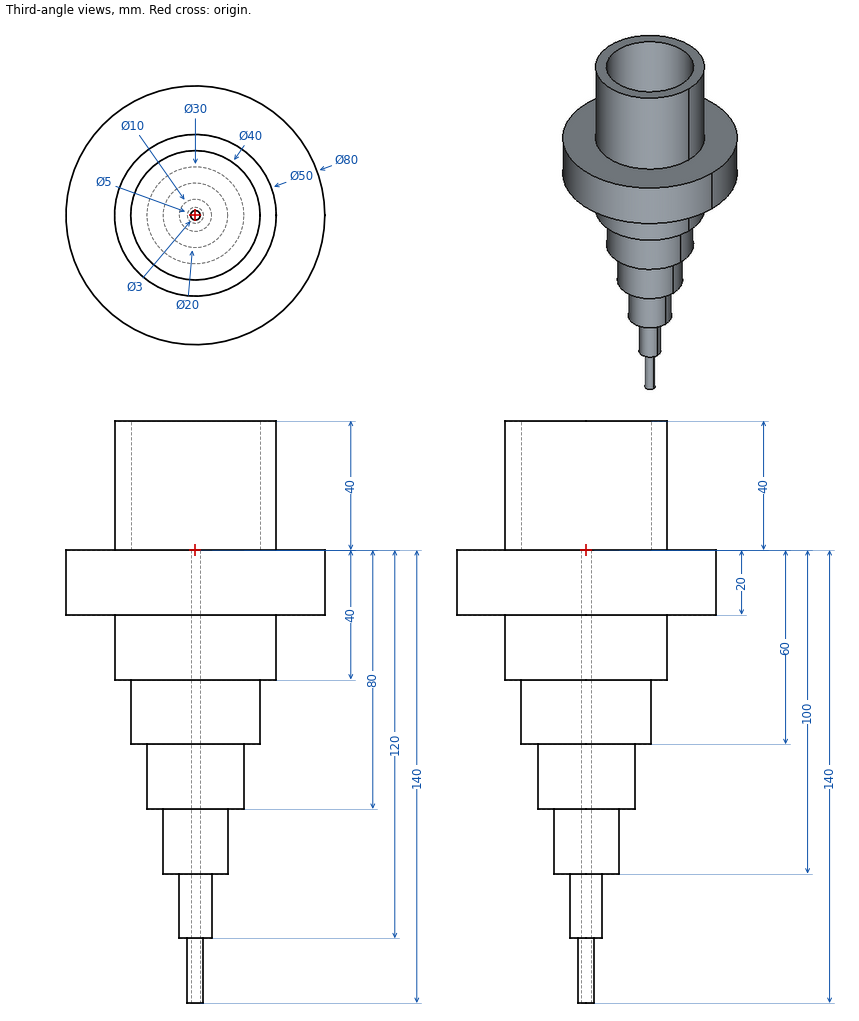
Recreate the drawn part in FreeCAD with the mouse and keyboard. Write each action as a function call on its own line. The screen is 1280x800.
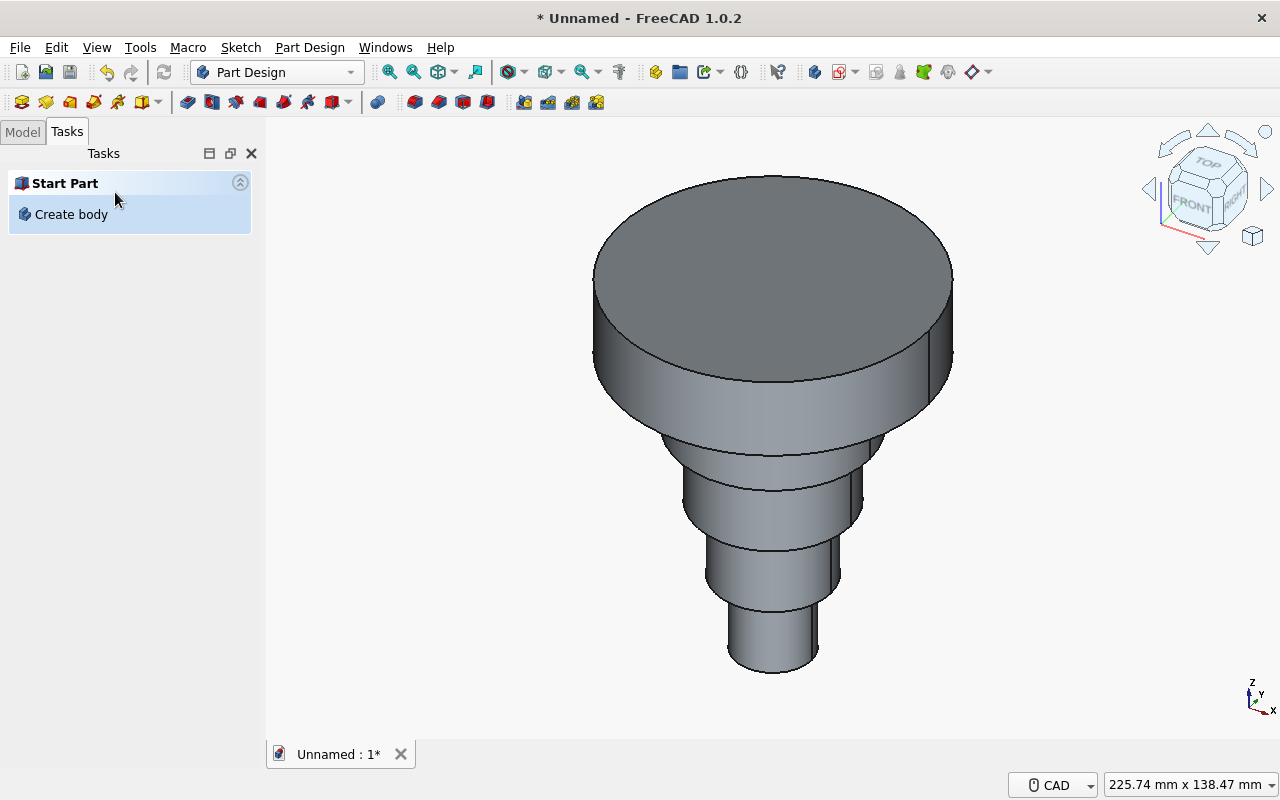
key(v)
key(f)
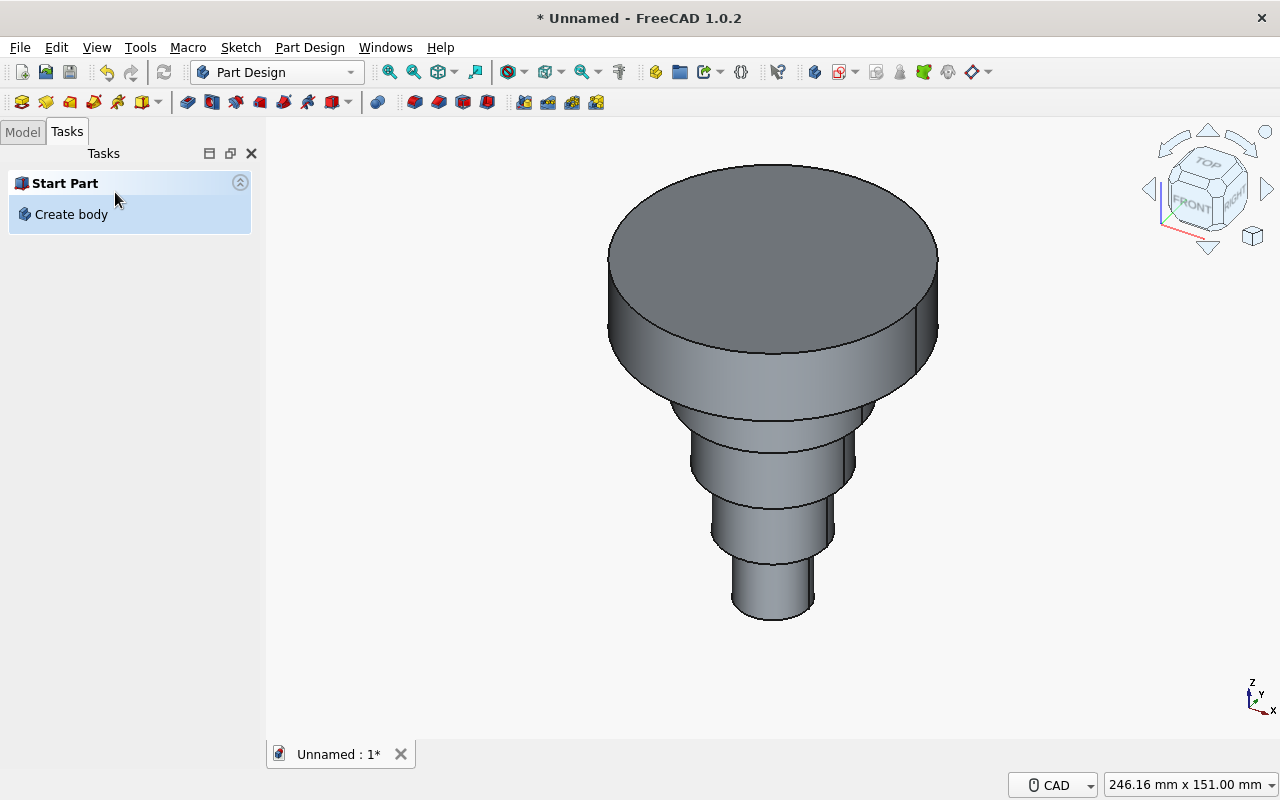
click(840, 72)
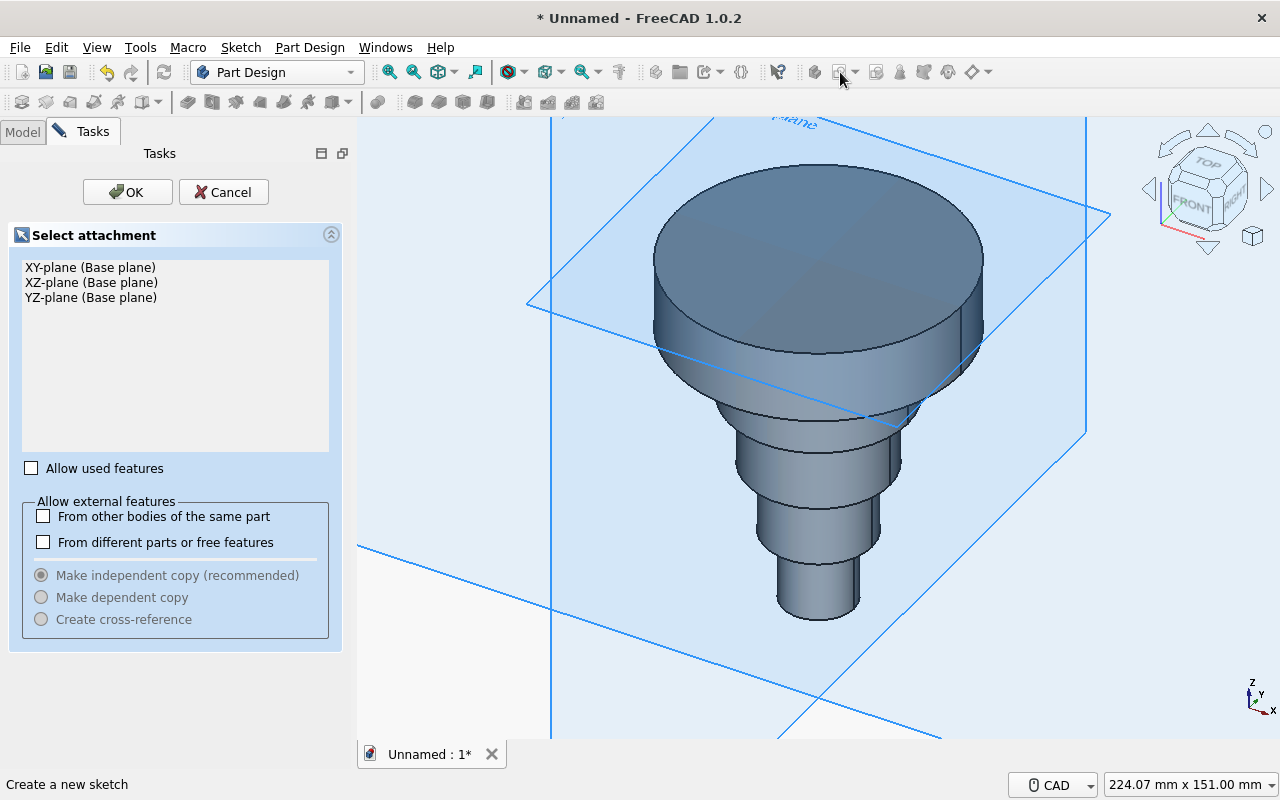
click(82, 268)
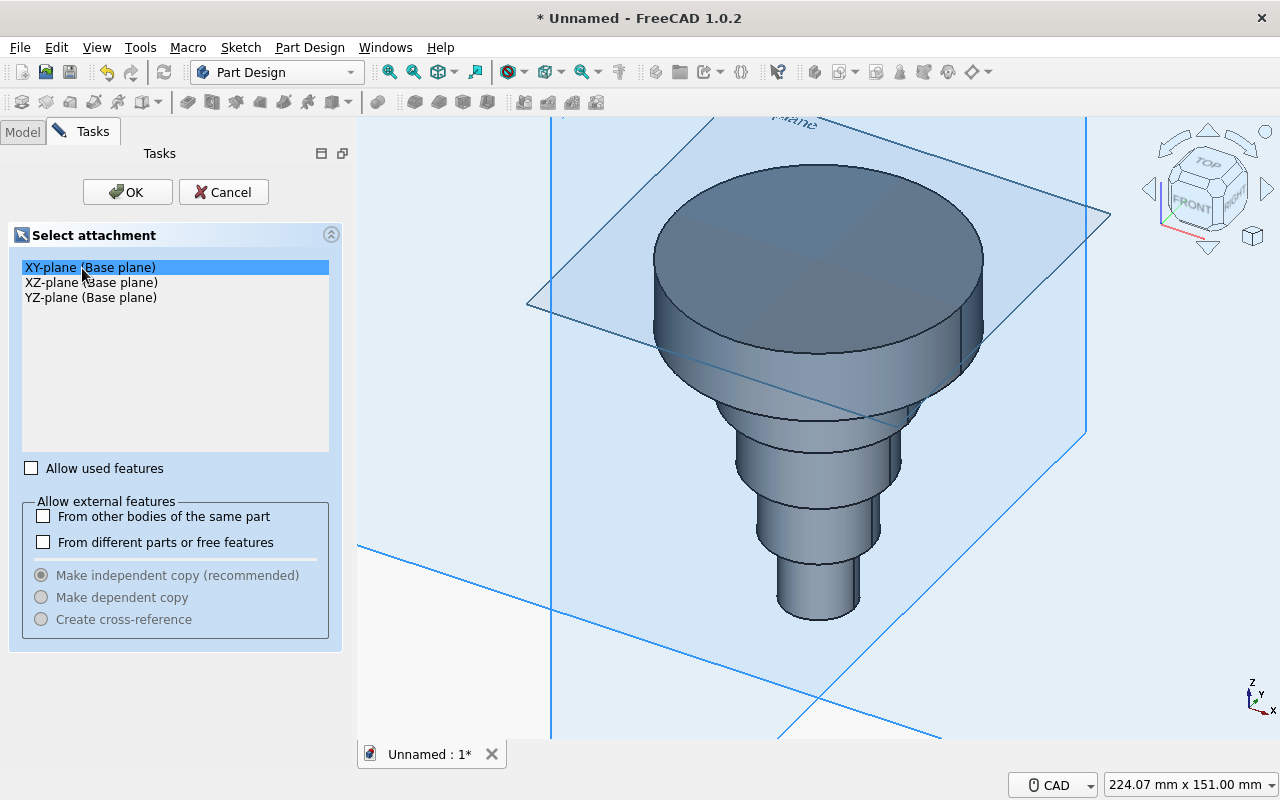
click(128, 192)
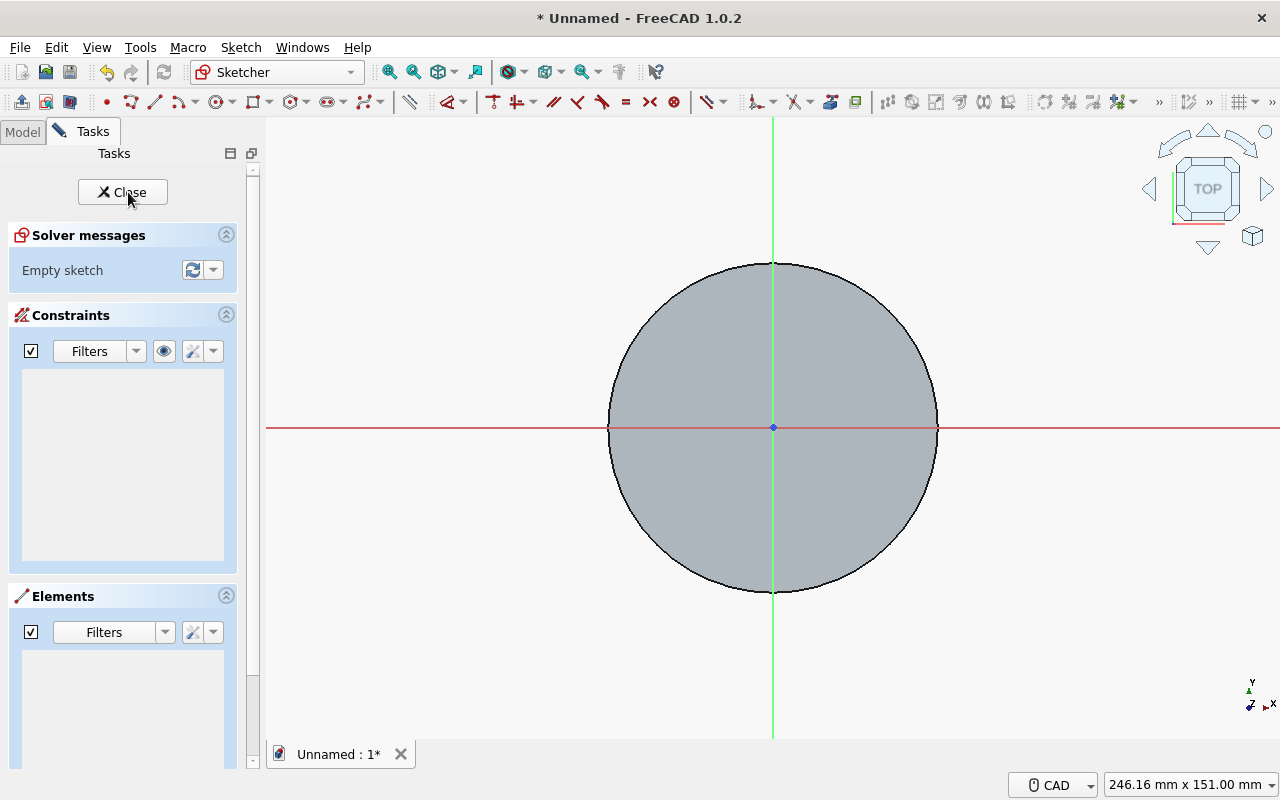
scroll(782, 428, up, 11)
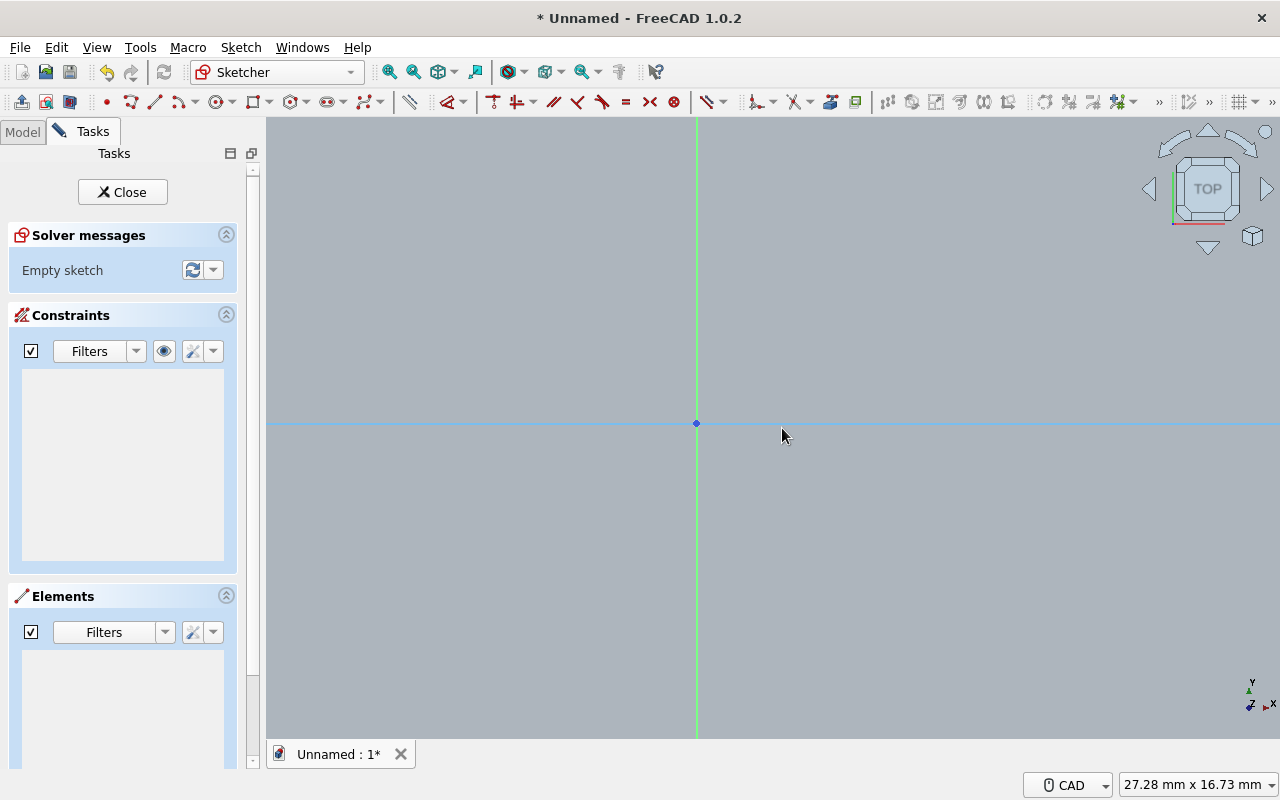
key(g)
key(c)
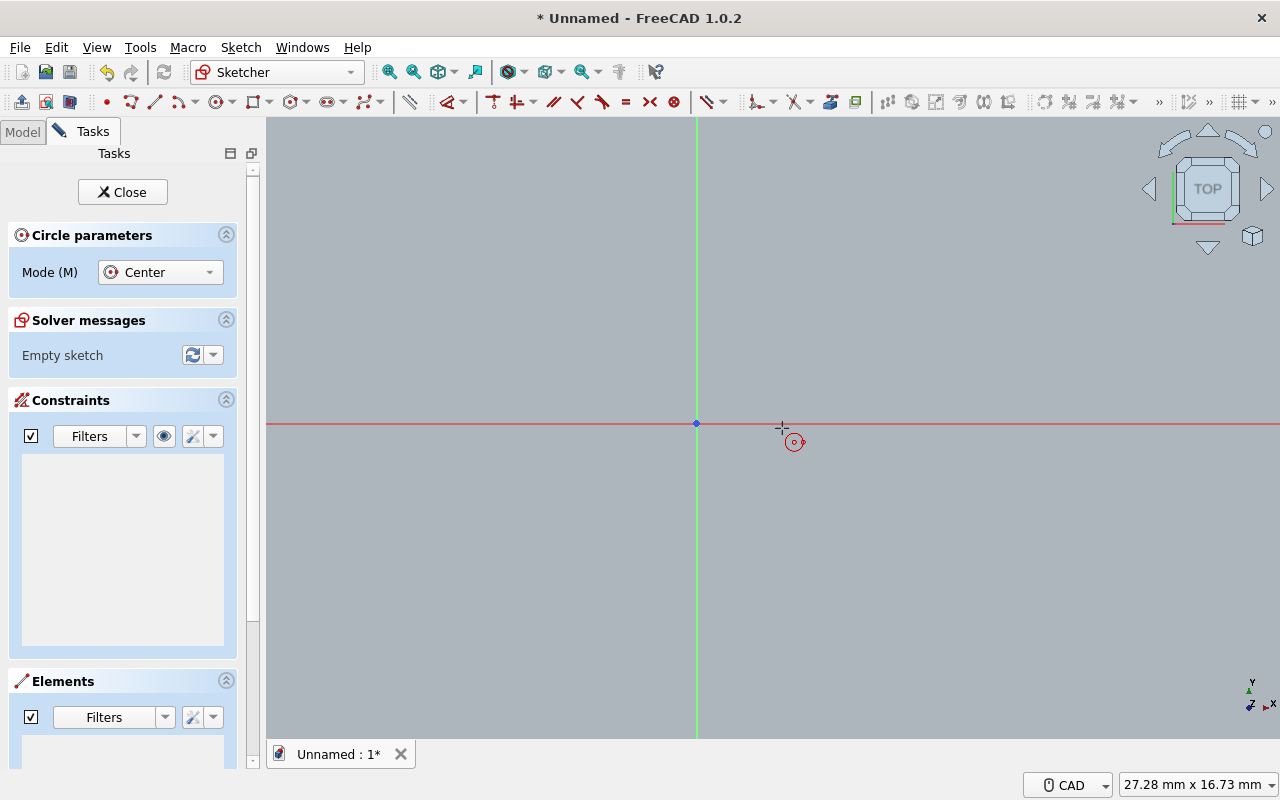
click(697, 424)
move(828, 293)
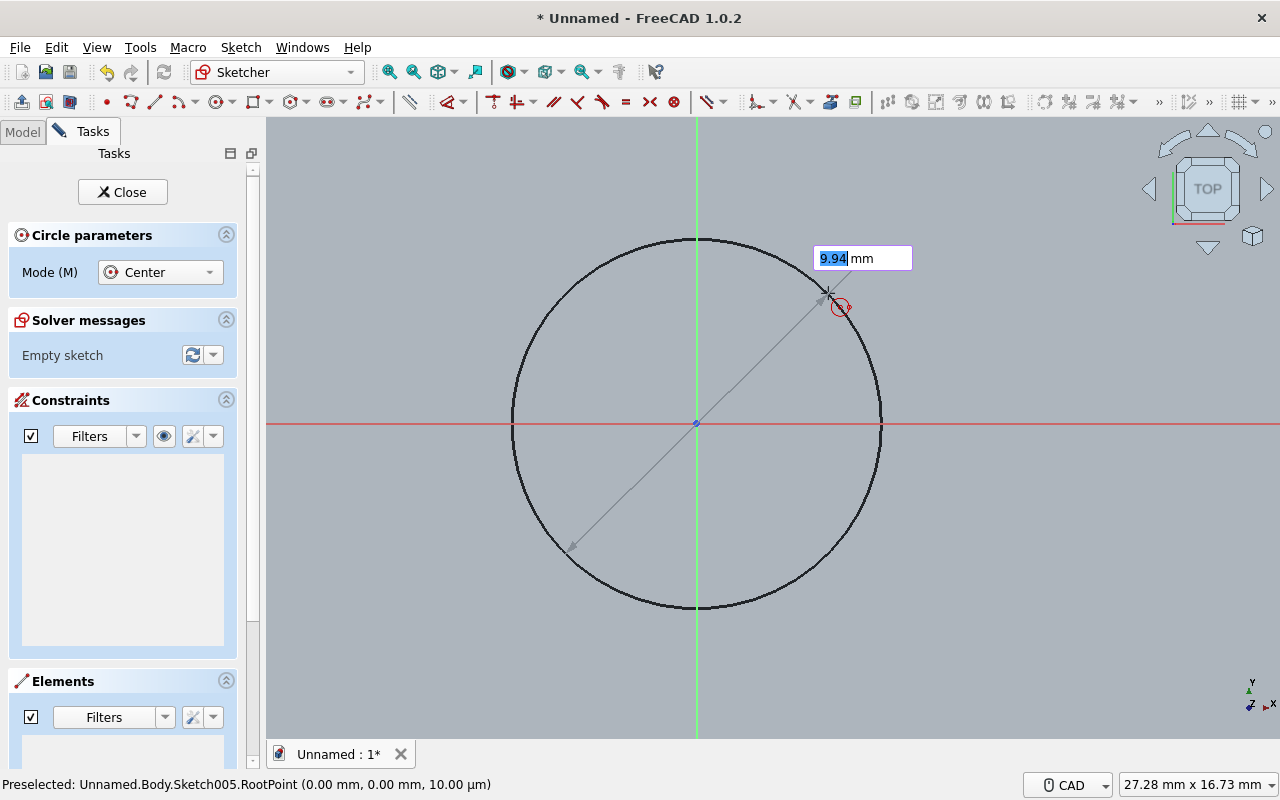
text(10)
key(Return)
key(Escape)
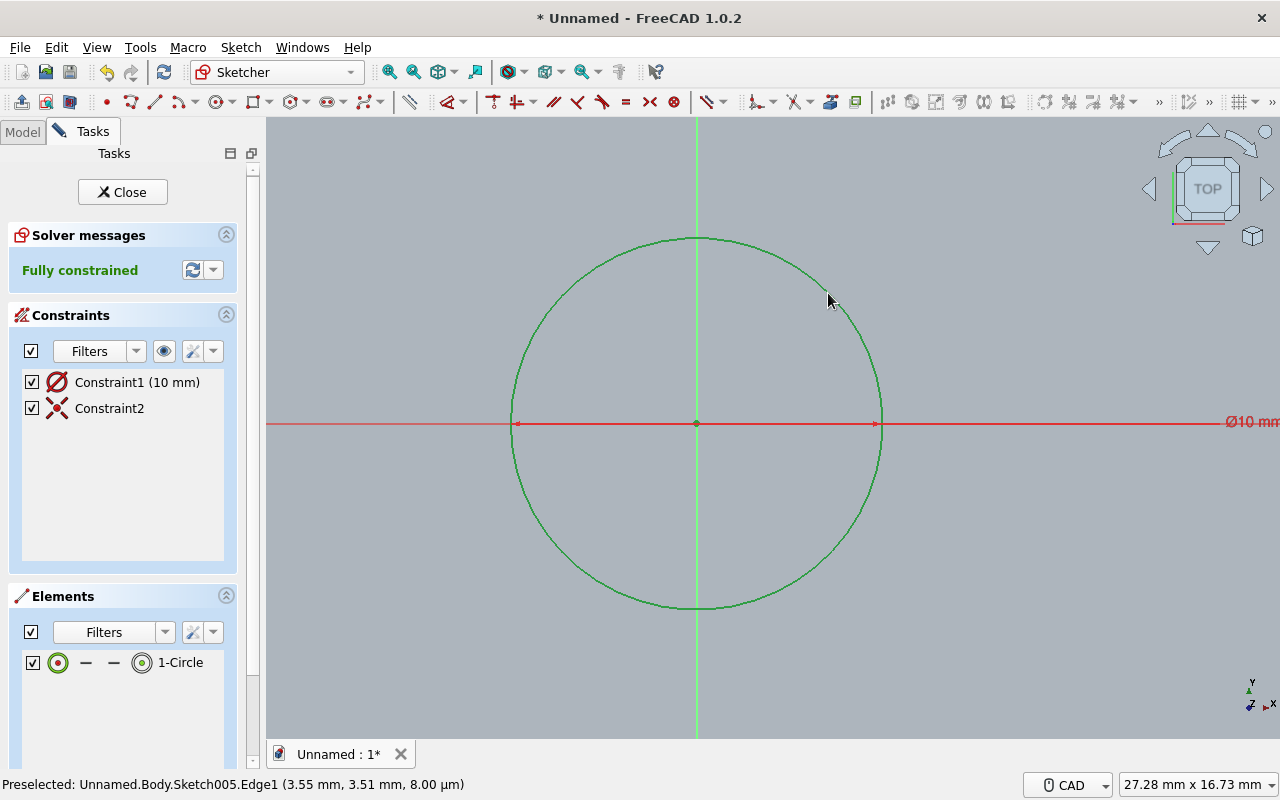
click(123, 192)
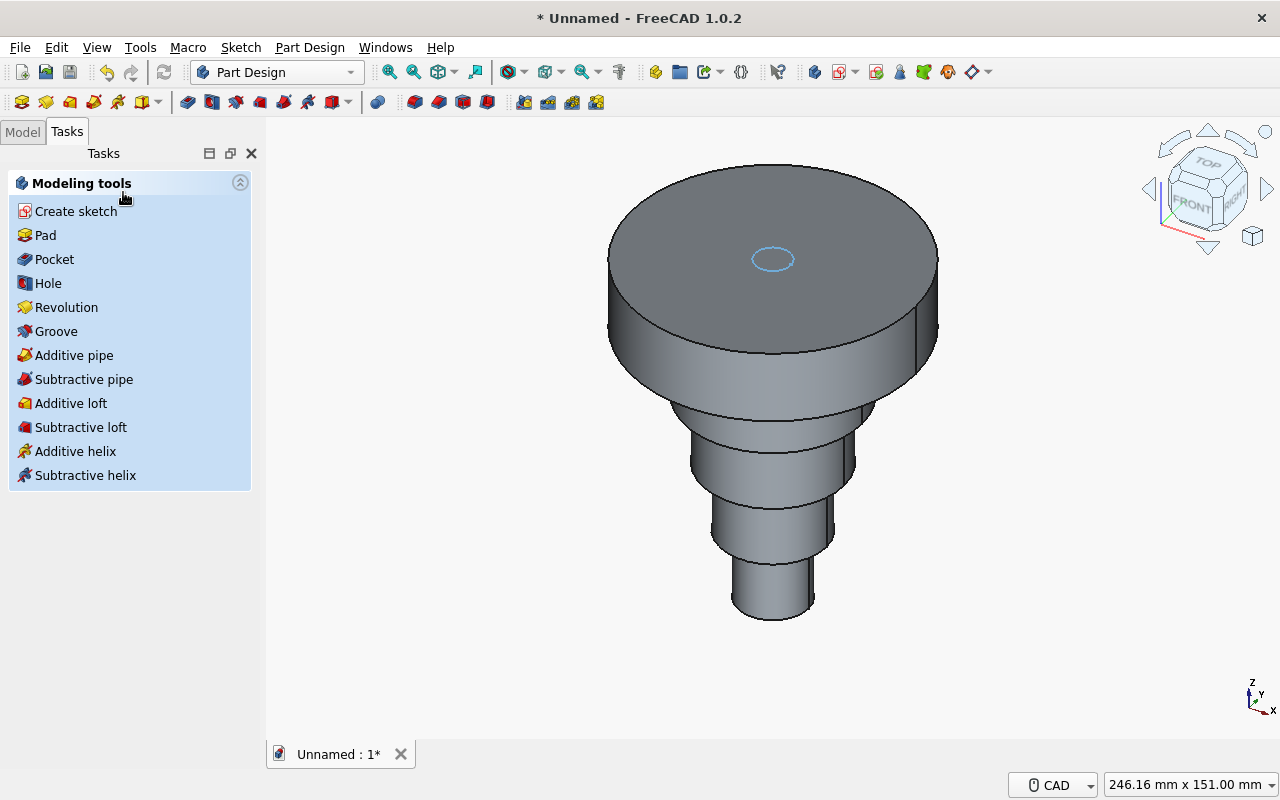
click(22, 102)